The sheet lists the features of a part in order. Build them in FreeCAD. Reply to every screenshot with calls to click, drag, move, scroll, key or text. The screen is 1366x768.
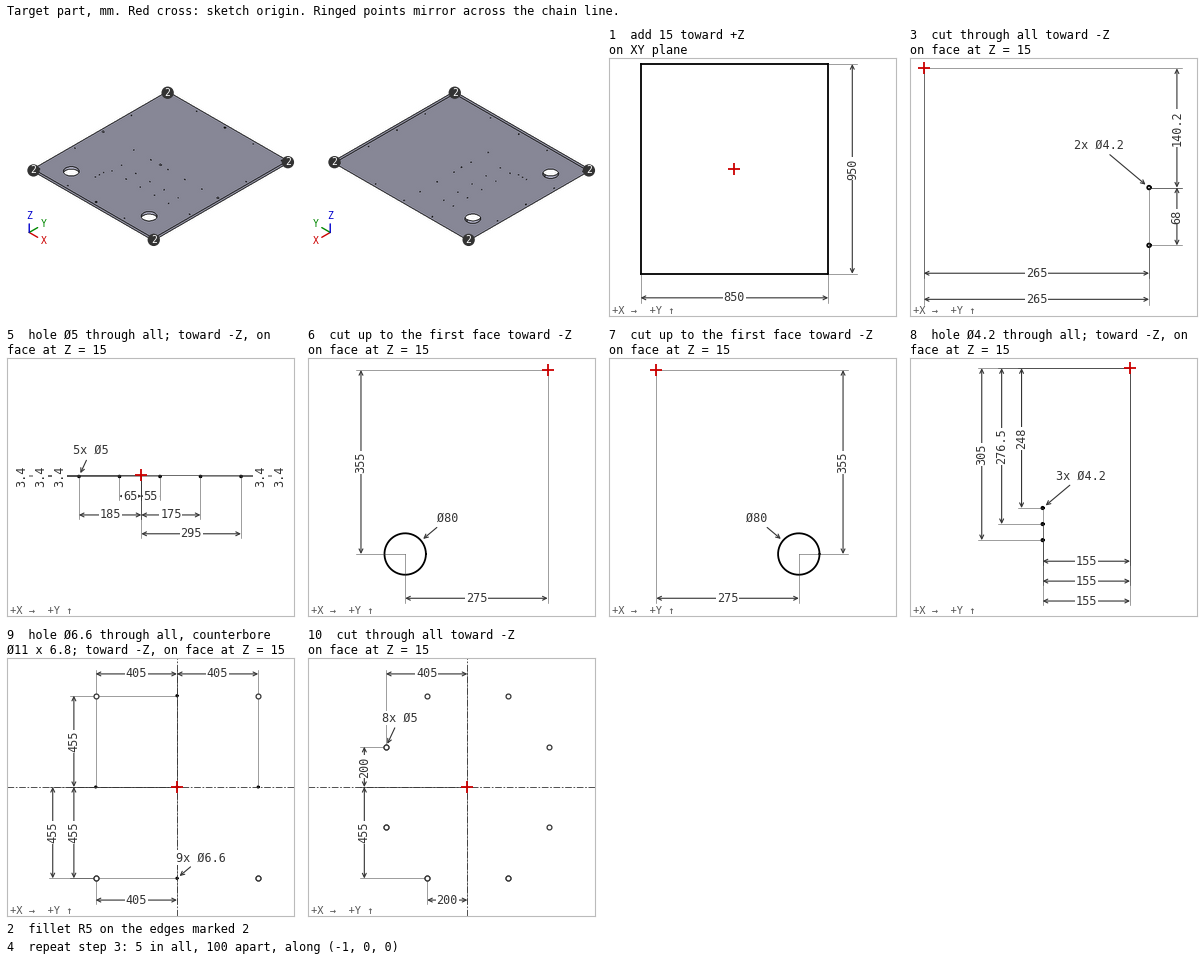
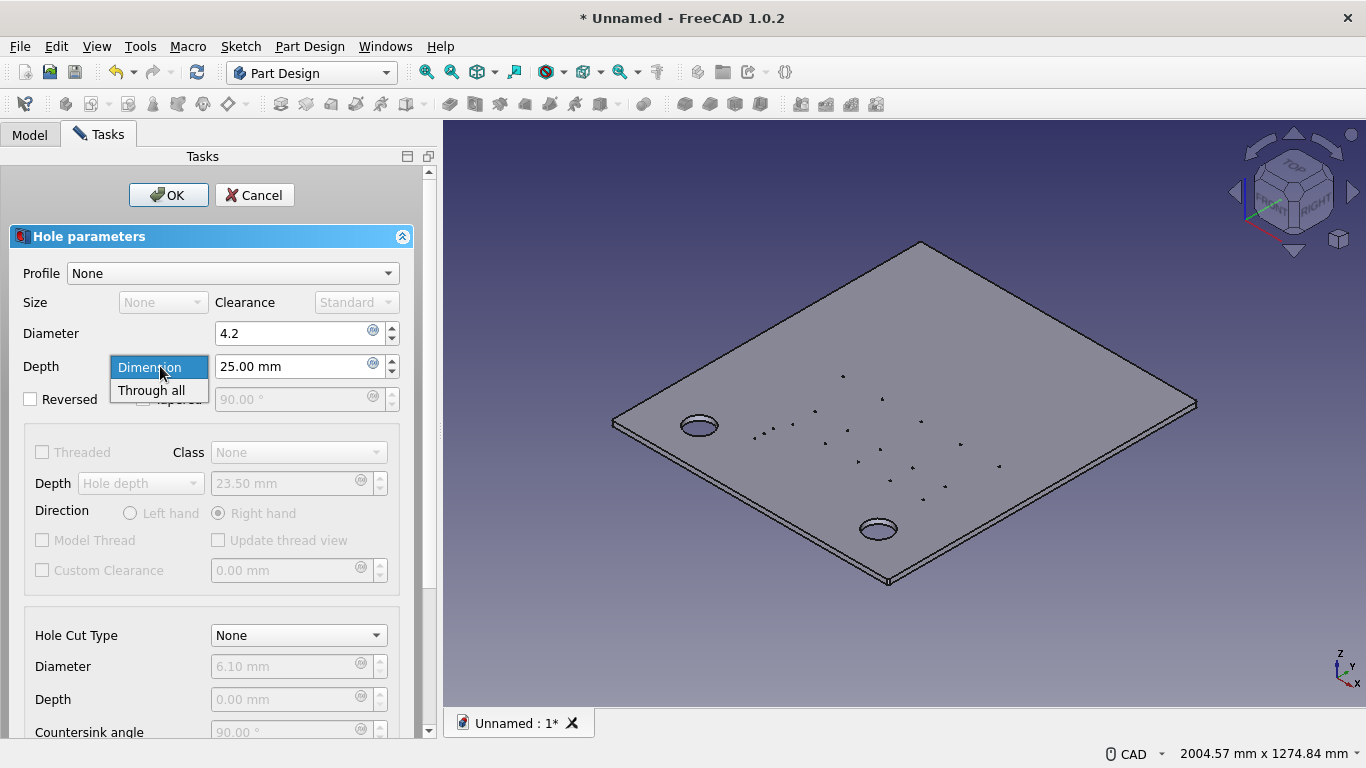
click(158, 390)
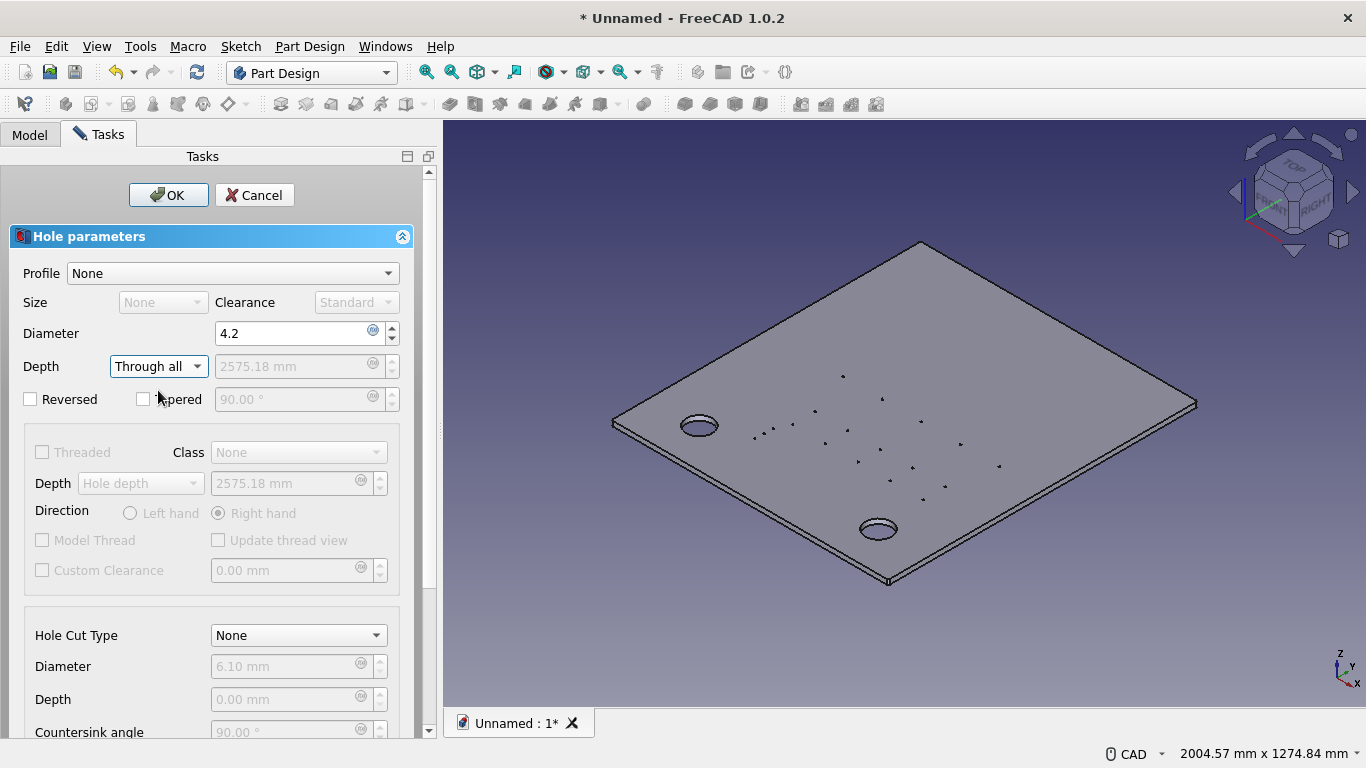
click(169, 195)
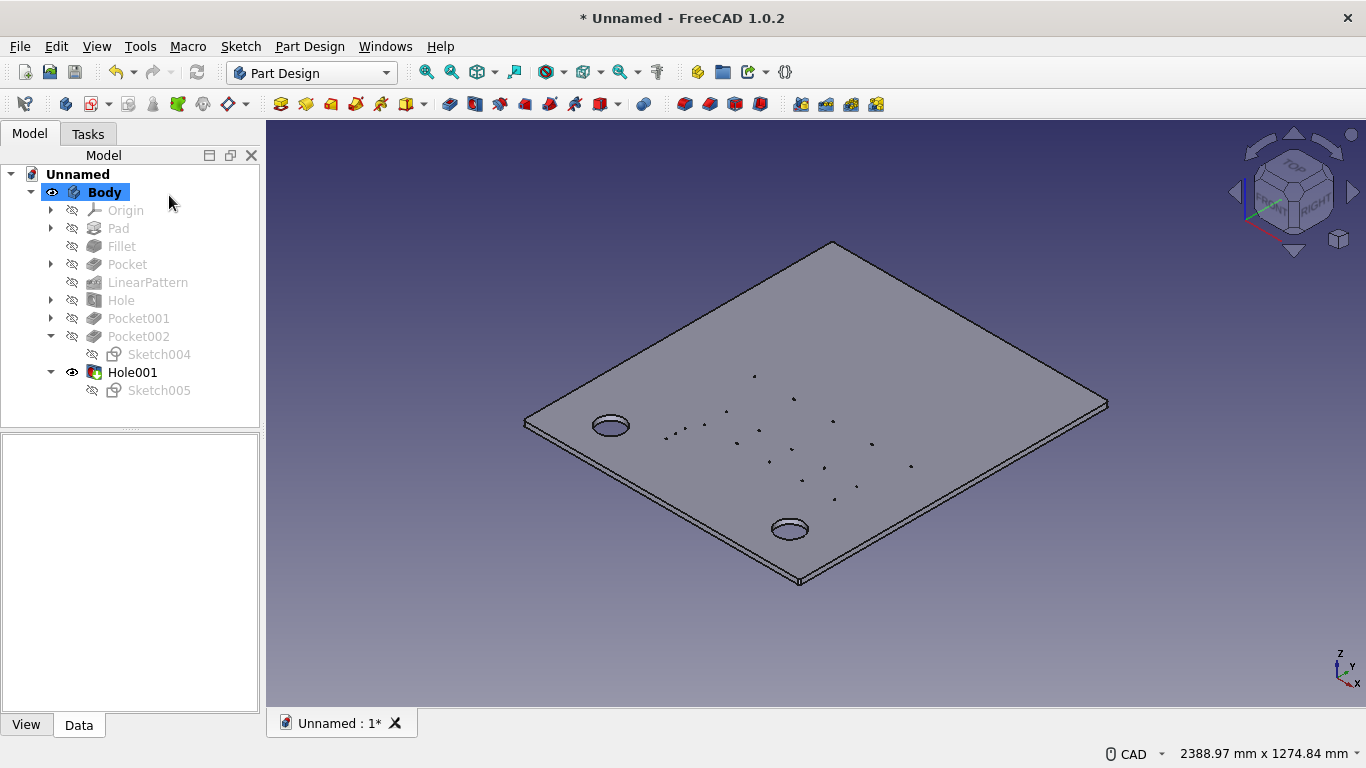
click(944, 381)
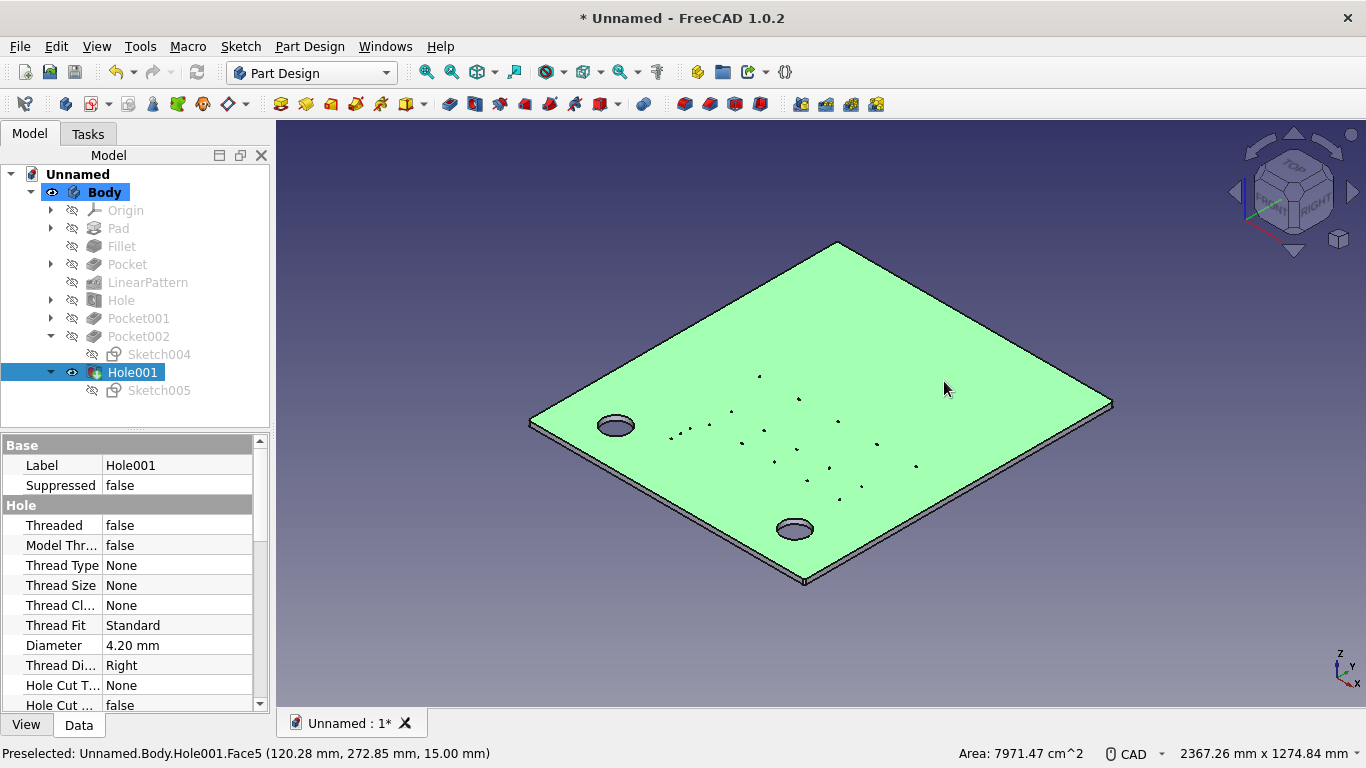
click(90, 104)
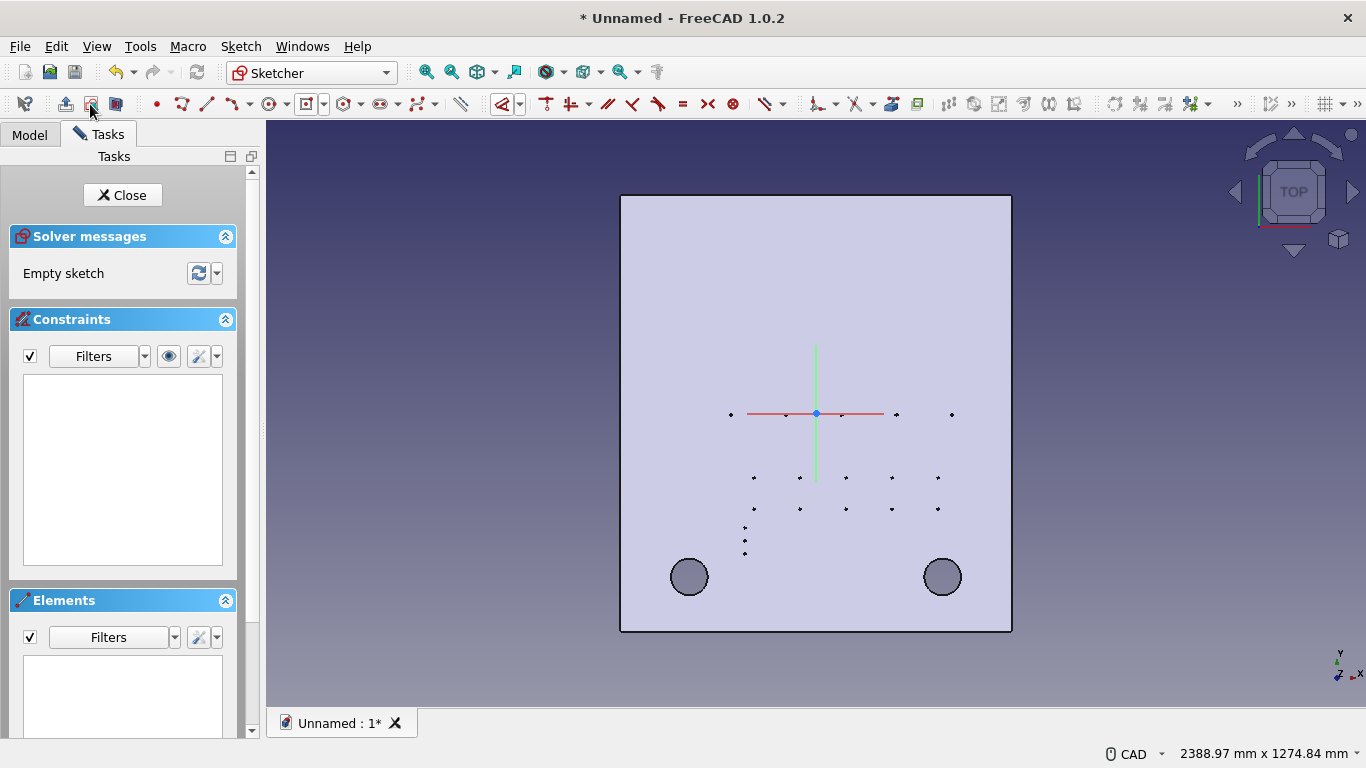
click(268, 104)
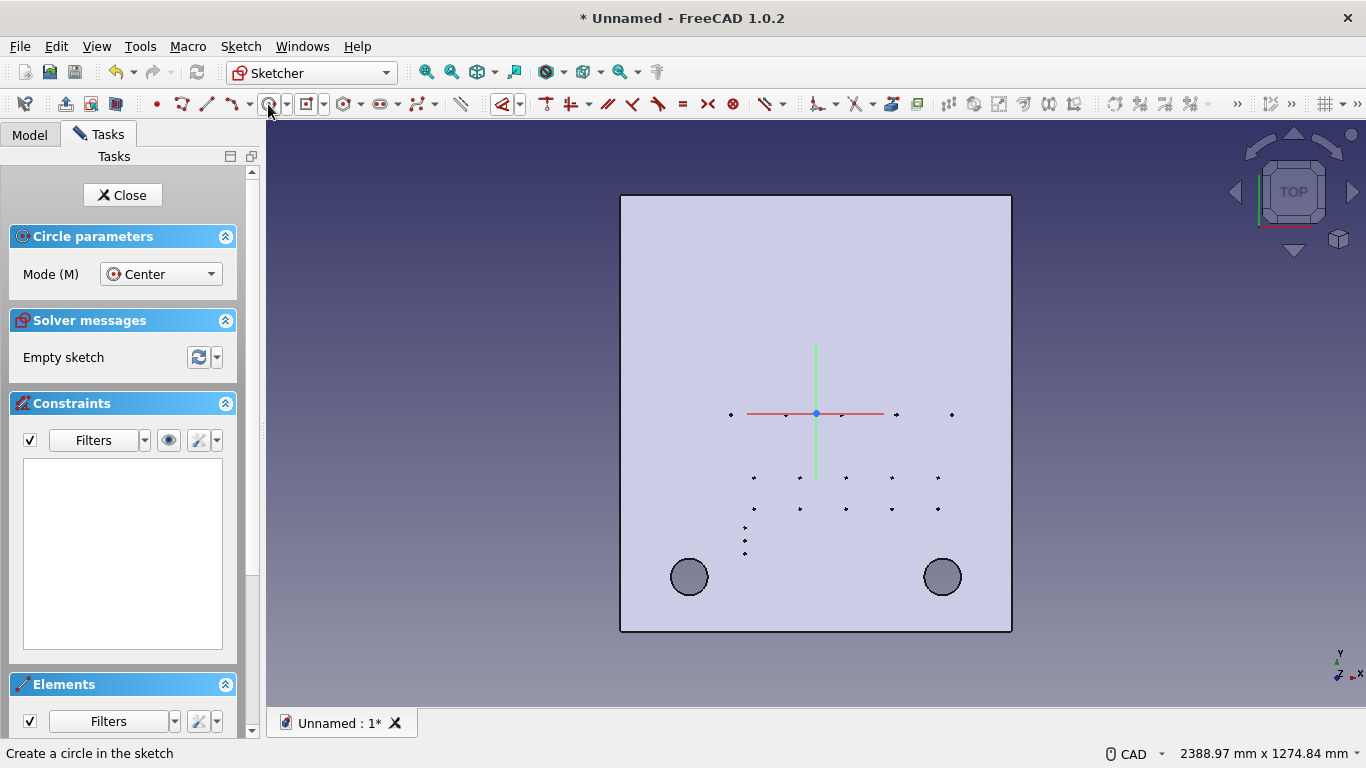
scroll(630, 623, up, 14)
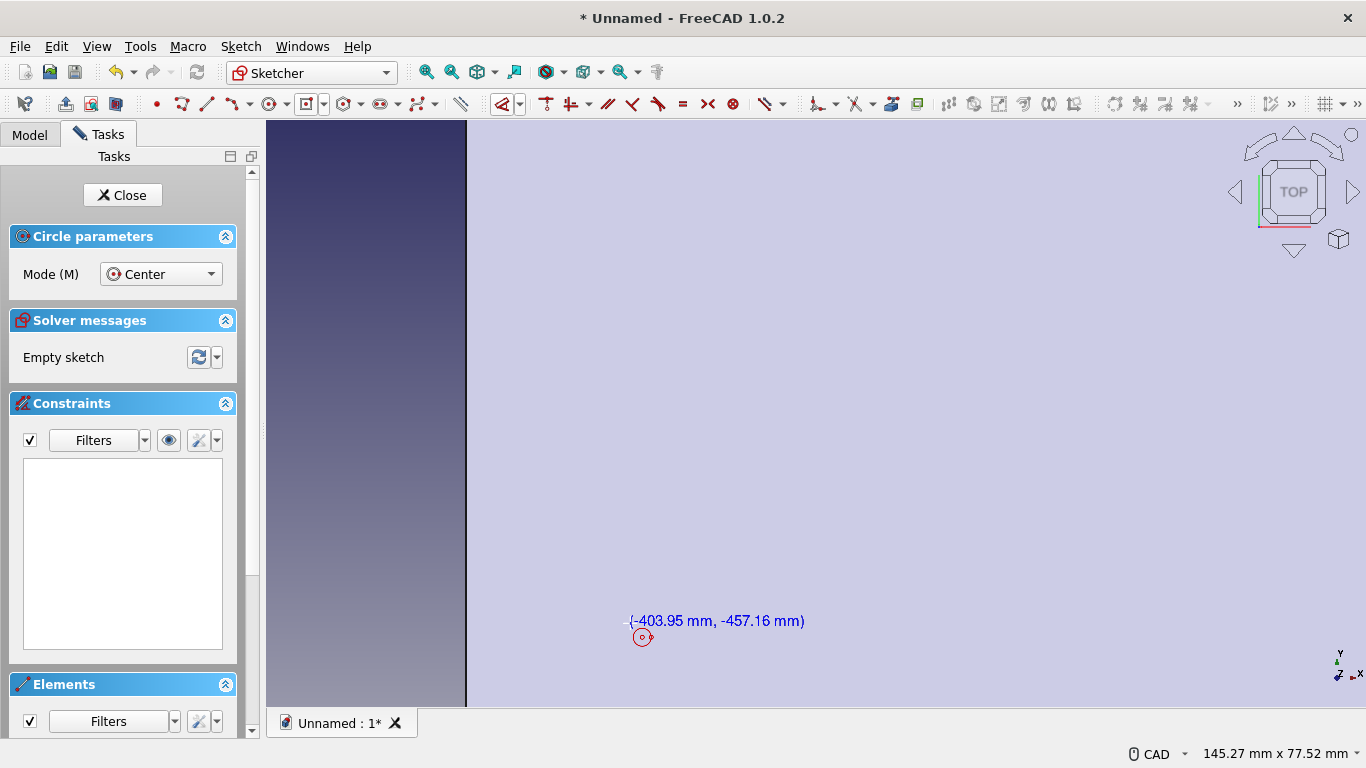
scroll(594, 584, down, 15)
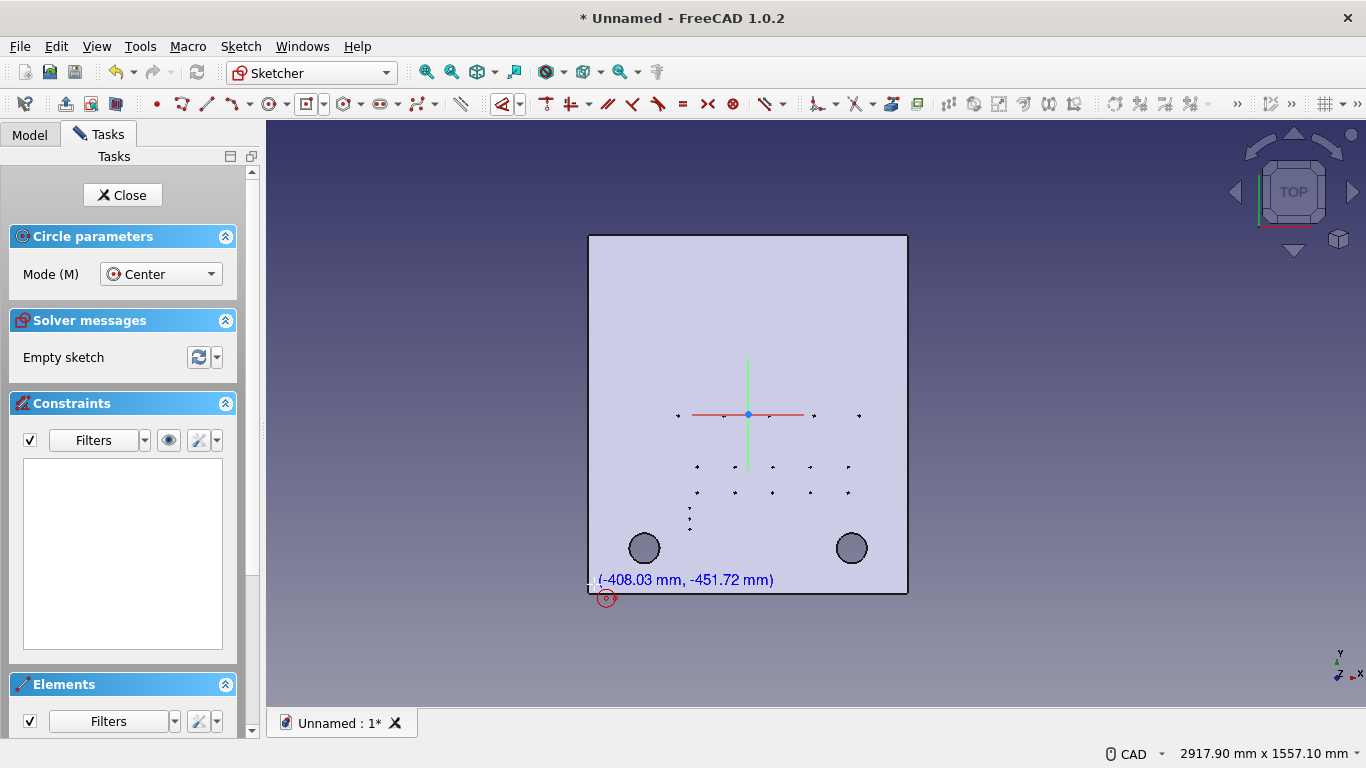
click(595, 586)
move(596, 585)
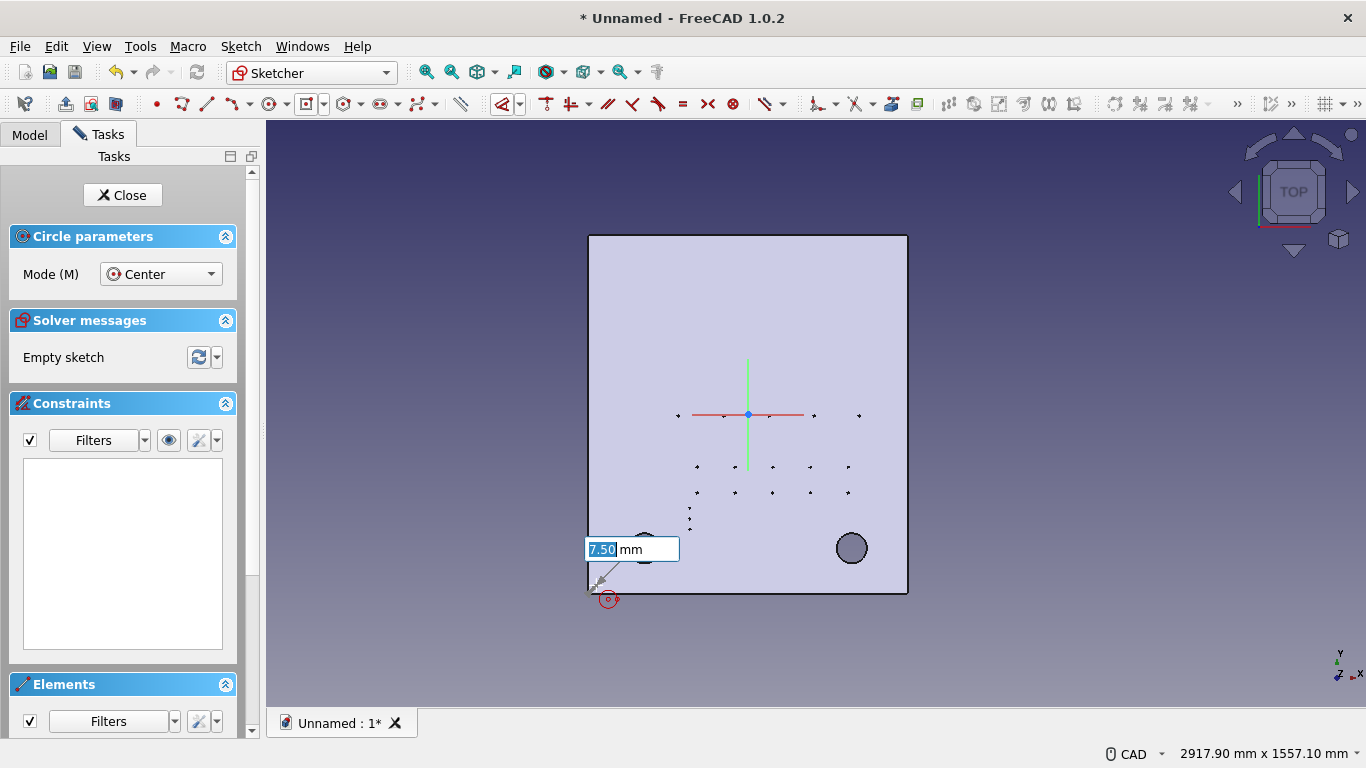
text(6.6)
key(Return)